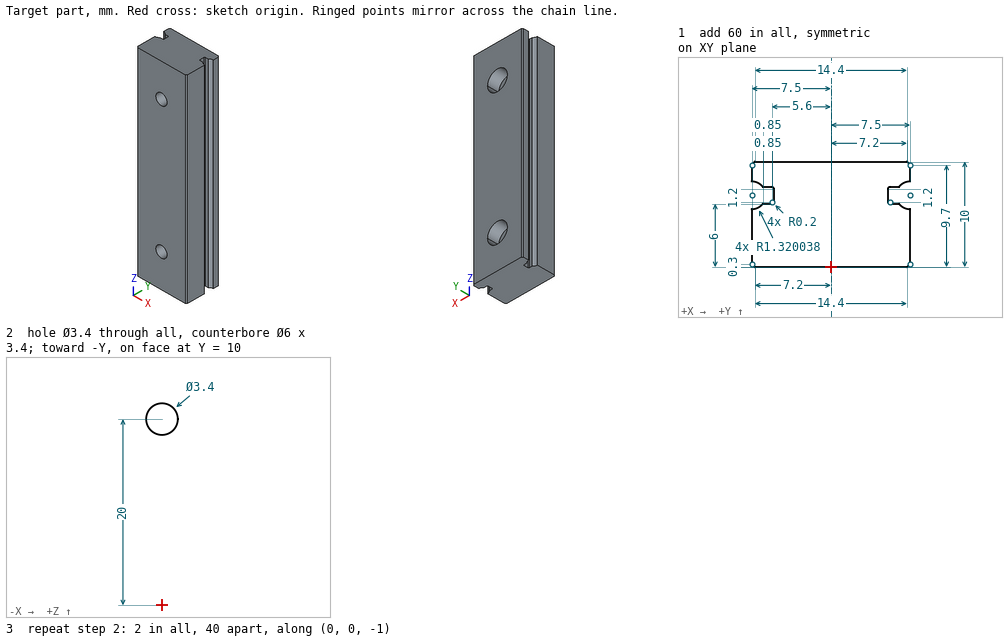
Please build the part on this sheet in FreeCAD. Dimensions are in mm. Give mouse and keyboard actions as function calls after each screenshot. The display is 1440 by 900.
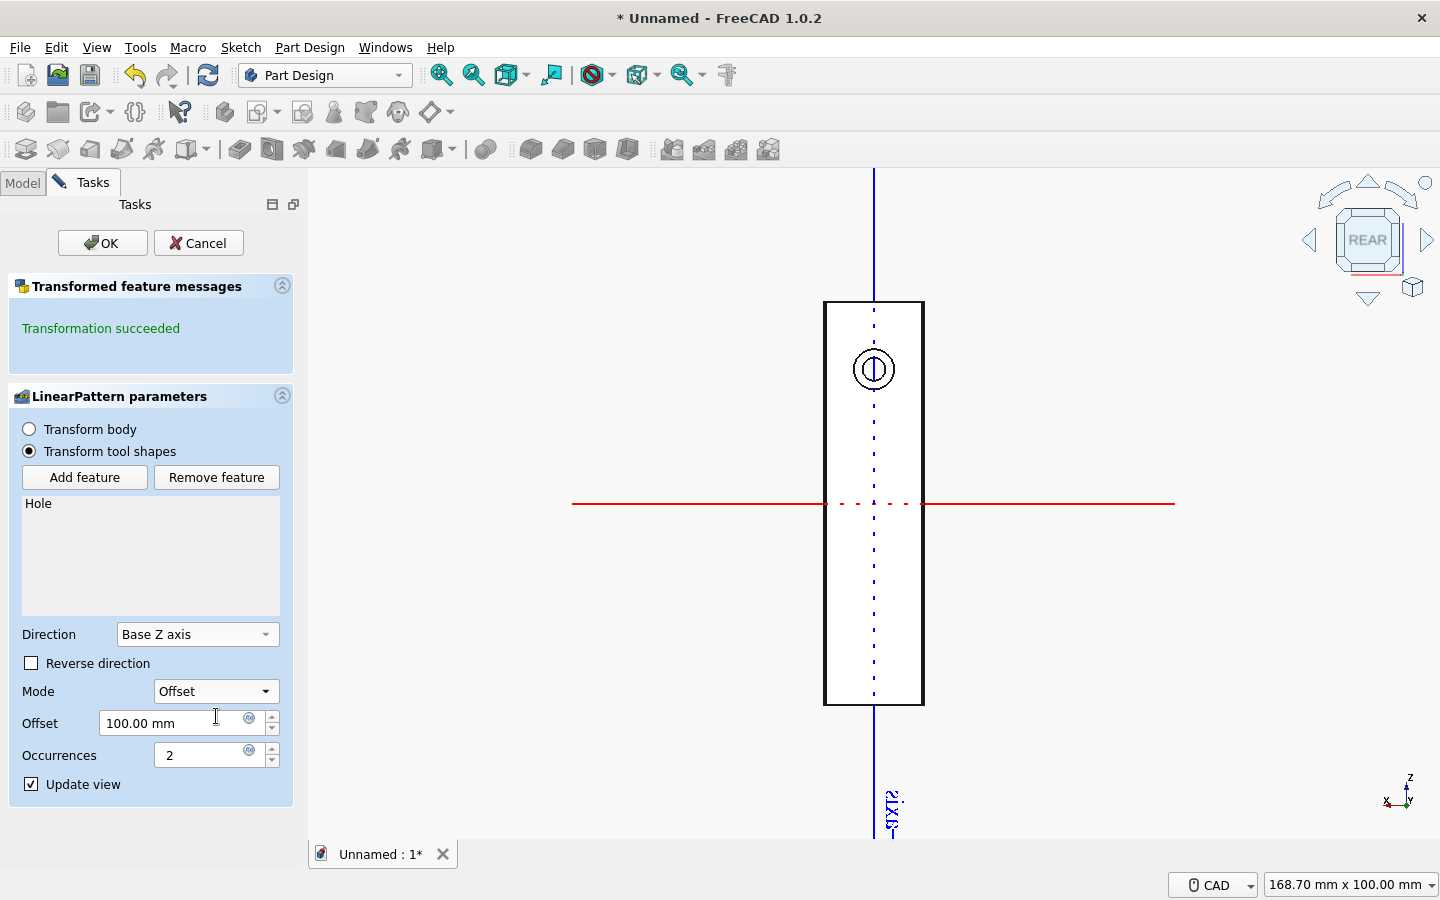
triple_click(182, 723)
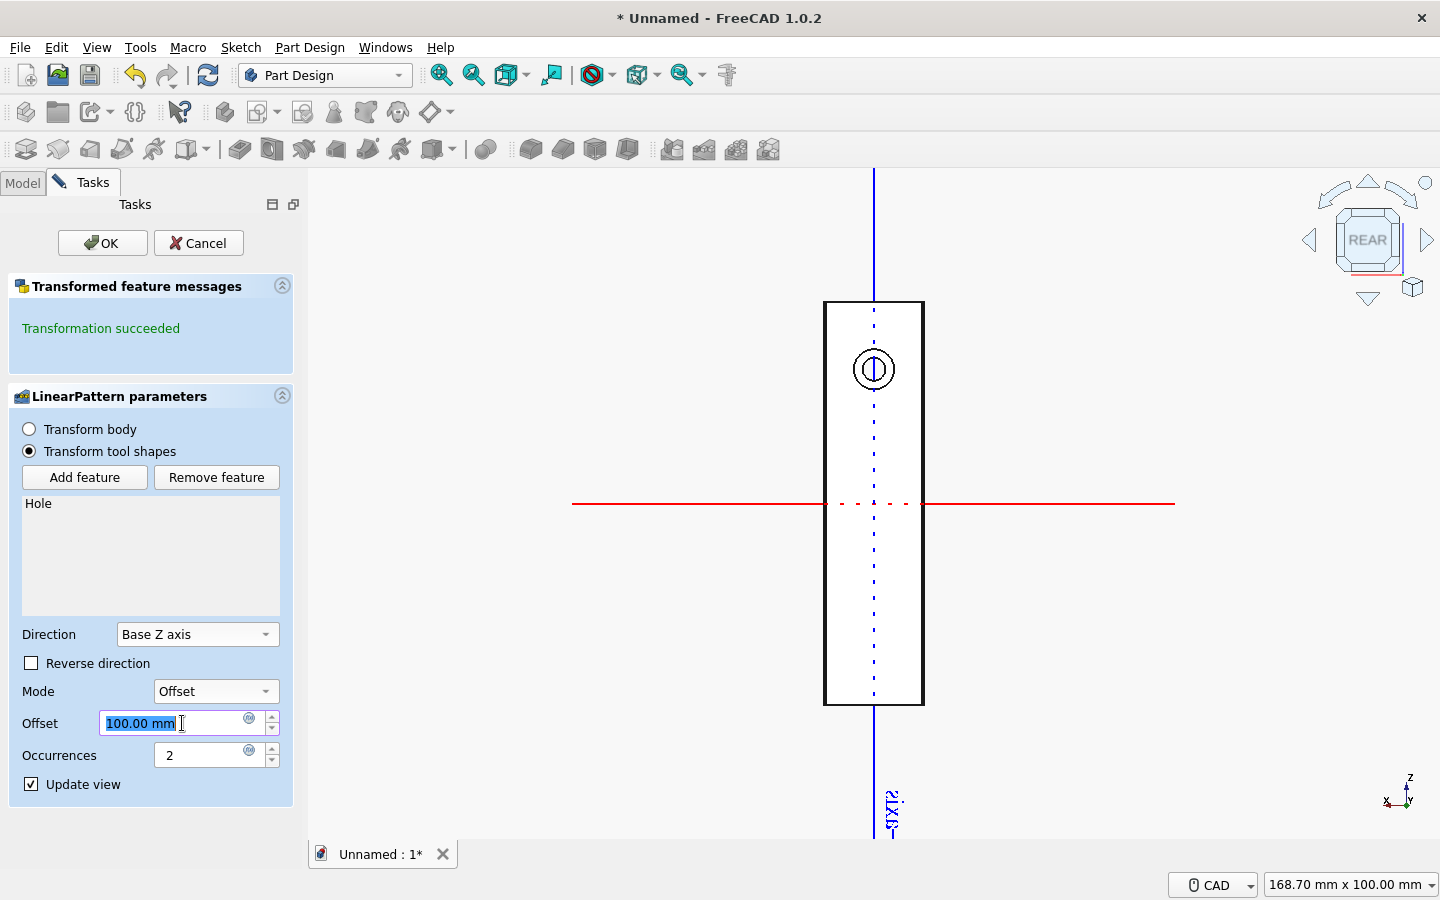
text(40)
key(Tab)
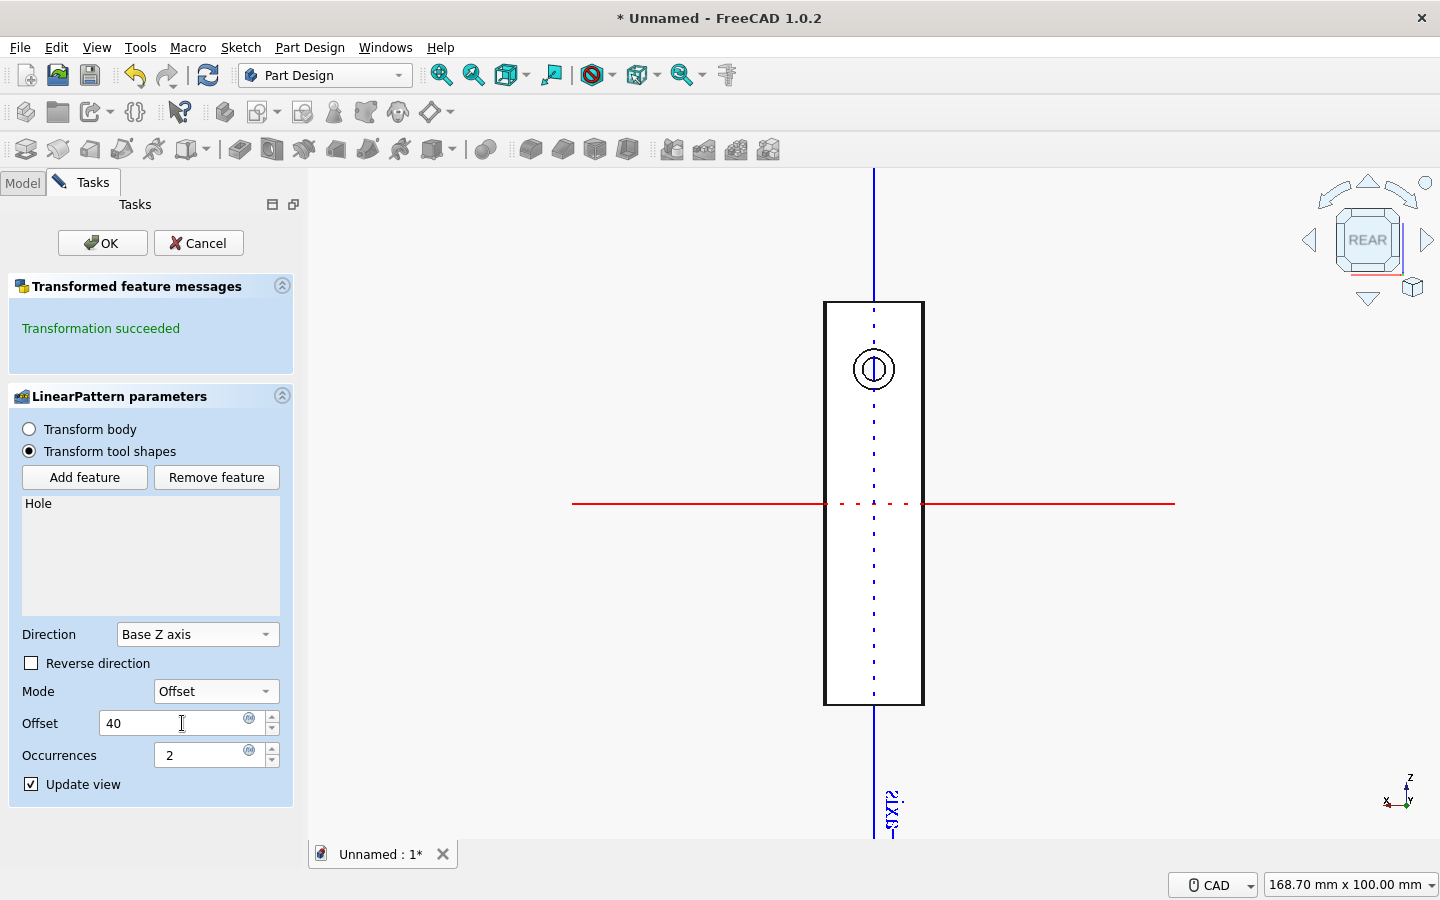
triple_click(209, 755)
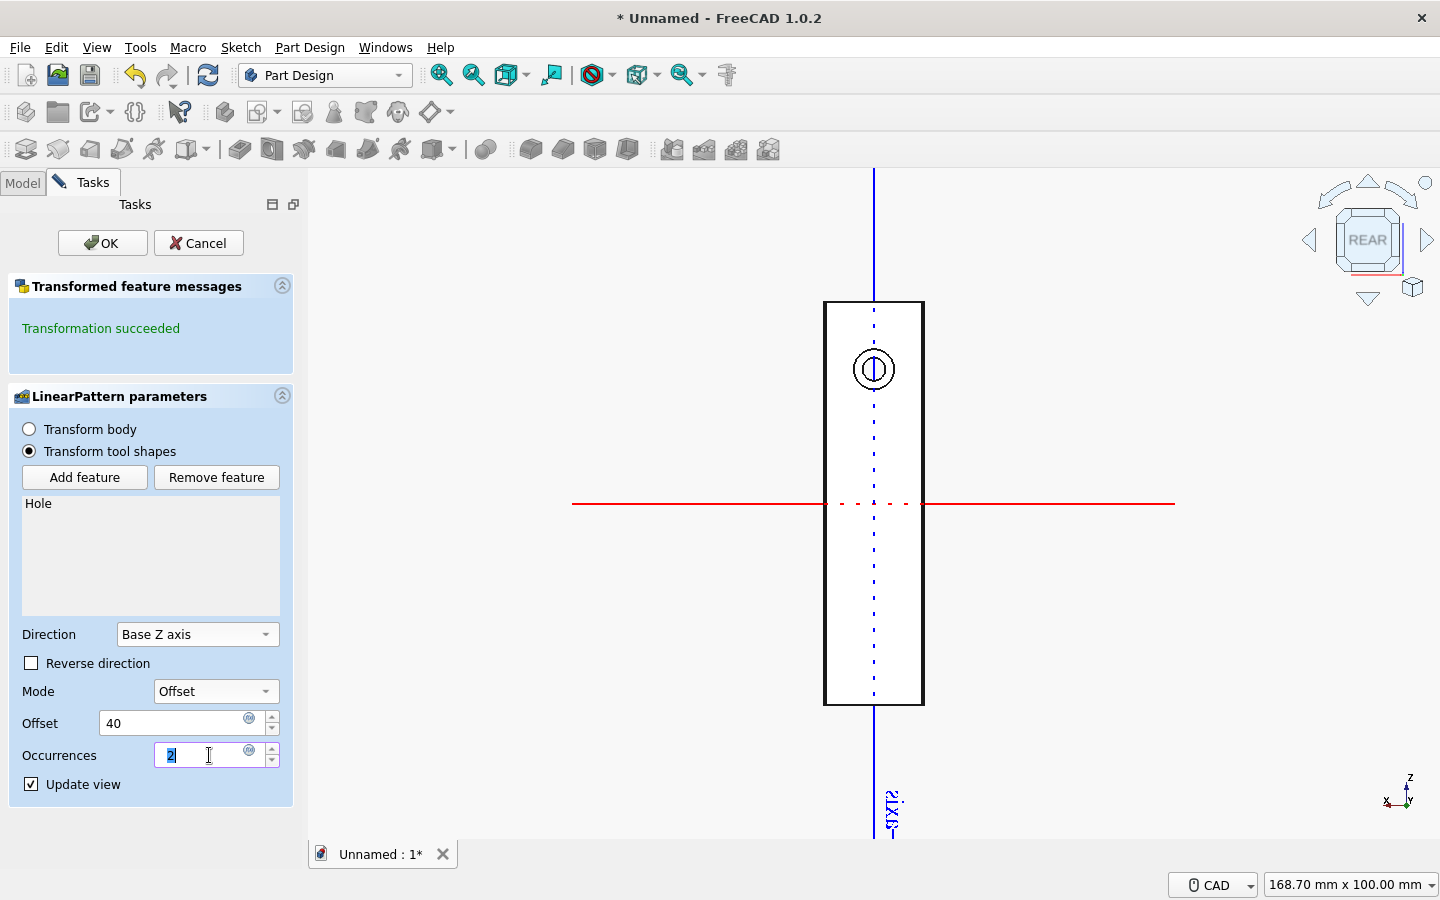
text(2)
key(Tab)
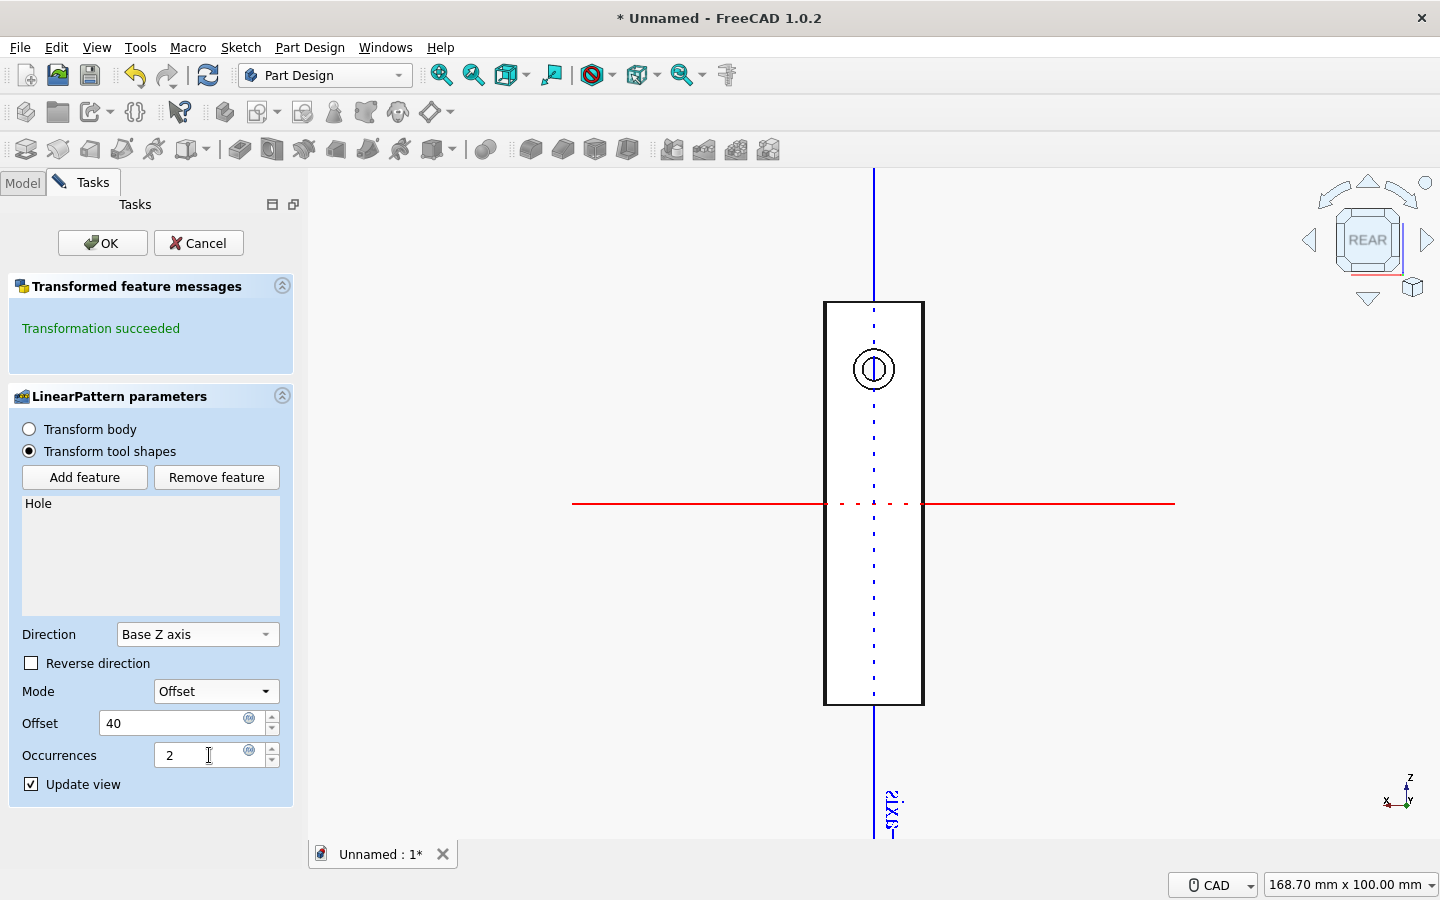
click(30, 663)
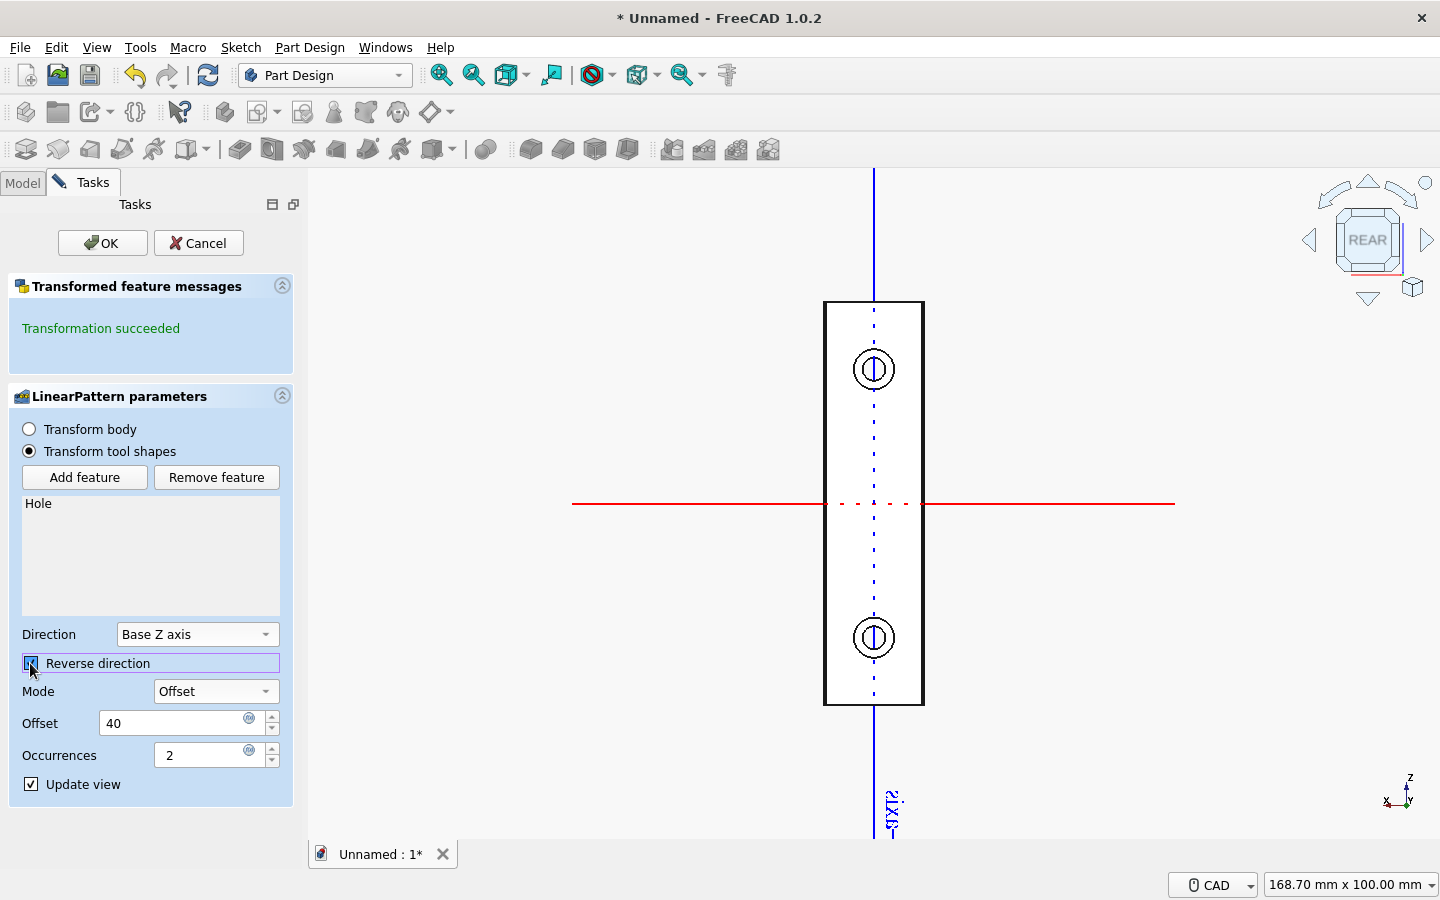
click(103, 243)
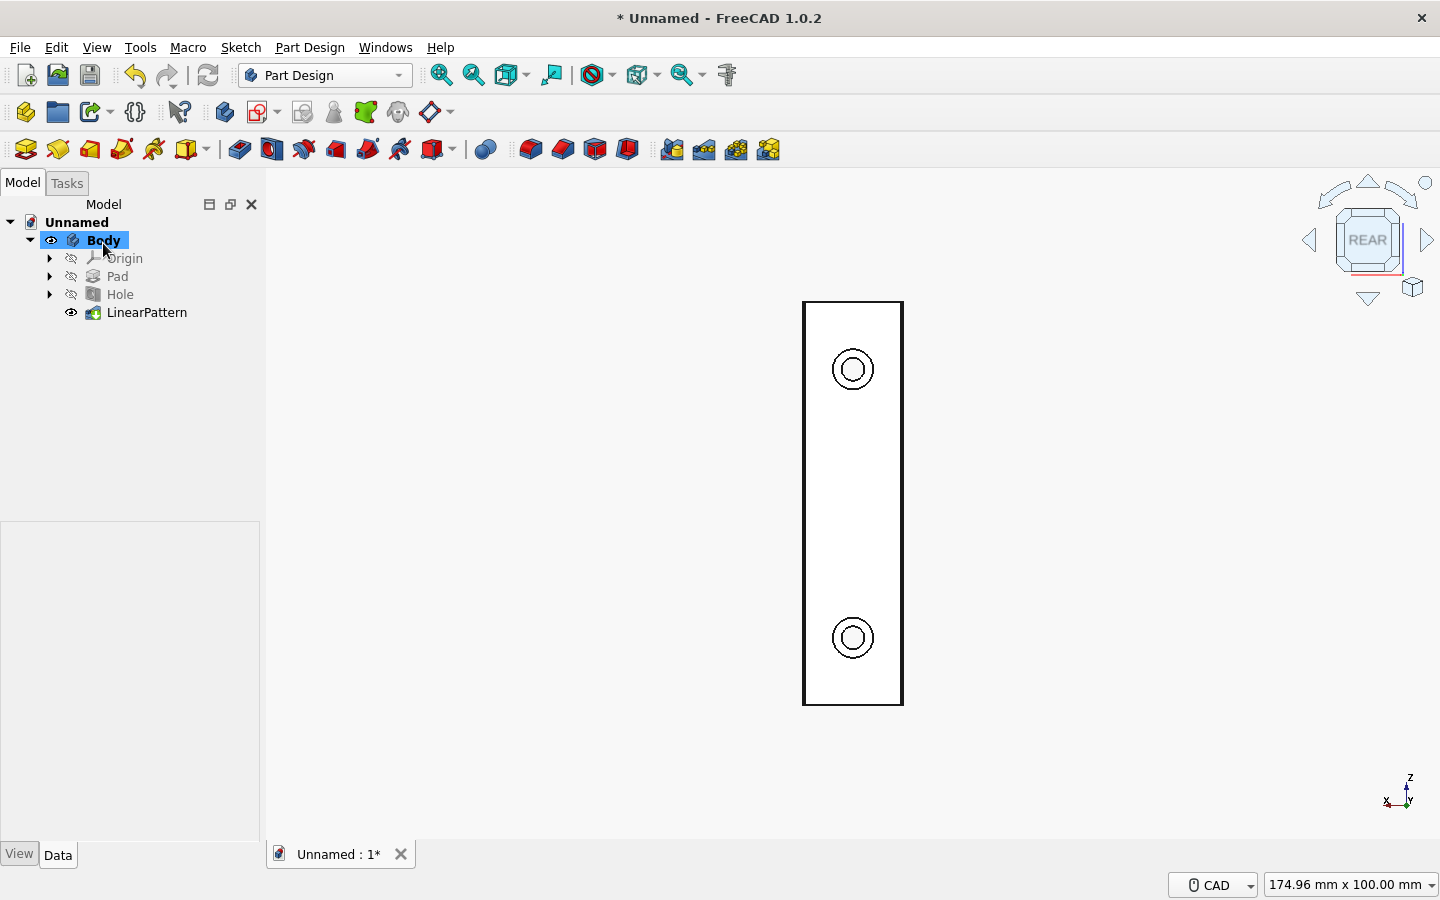
key(0)